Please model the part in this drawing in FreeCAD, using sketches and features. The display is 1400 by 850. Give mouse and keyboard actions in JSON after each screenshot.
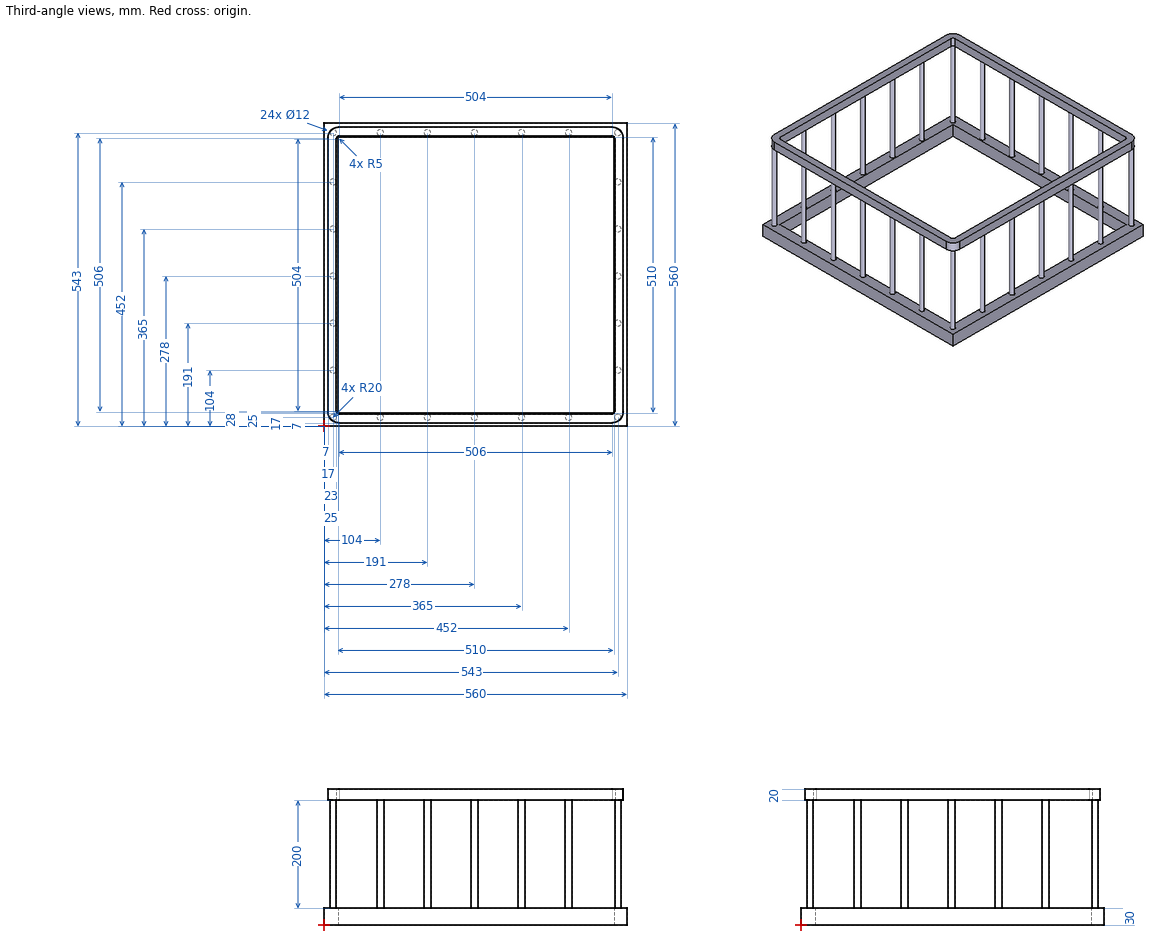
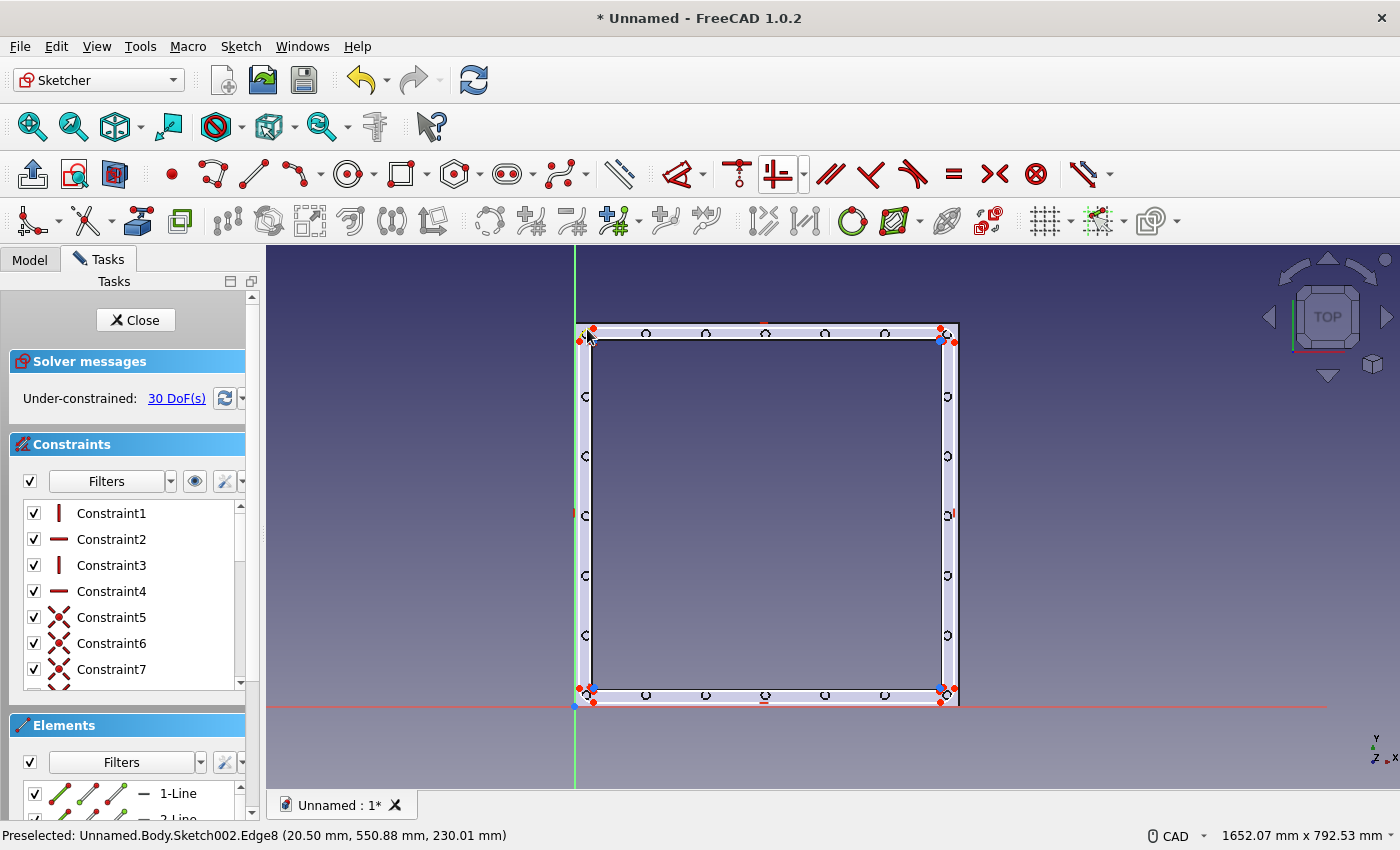
{"action": "scroll", "coordinate": [697, 703], "scroll_direction": "up", "scroll_amount": 6}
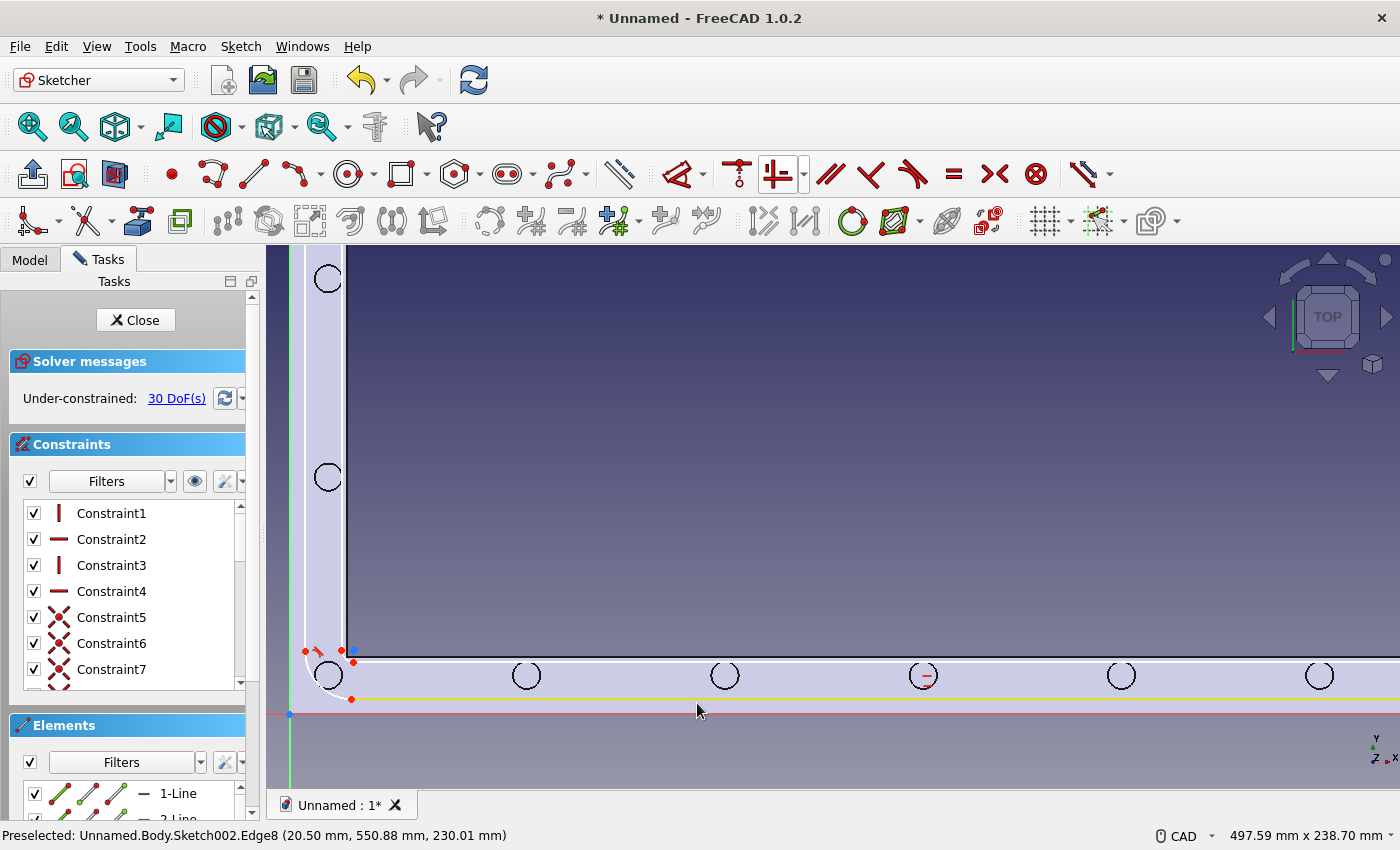
{"action": "left_click", "coordinate": [697, 699]}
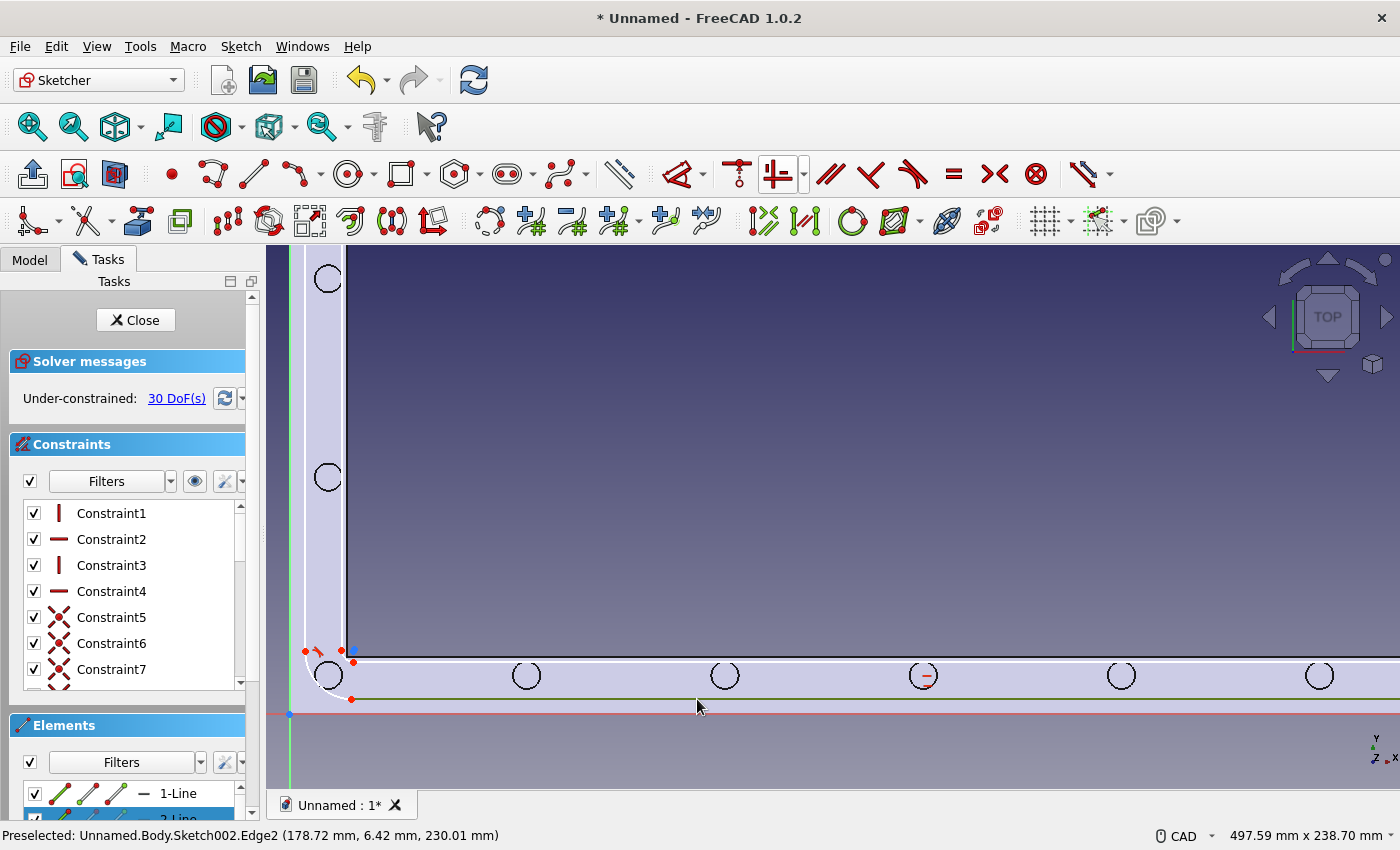
{"action": "left_click", "coordinate": [310, 673]}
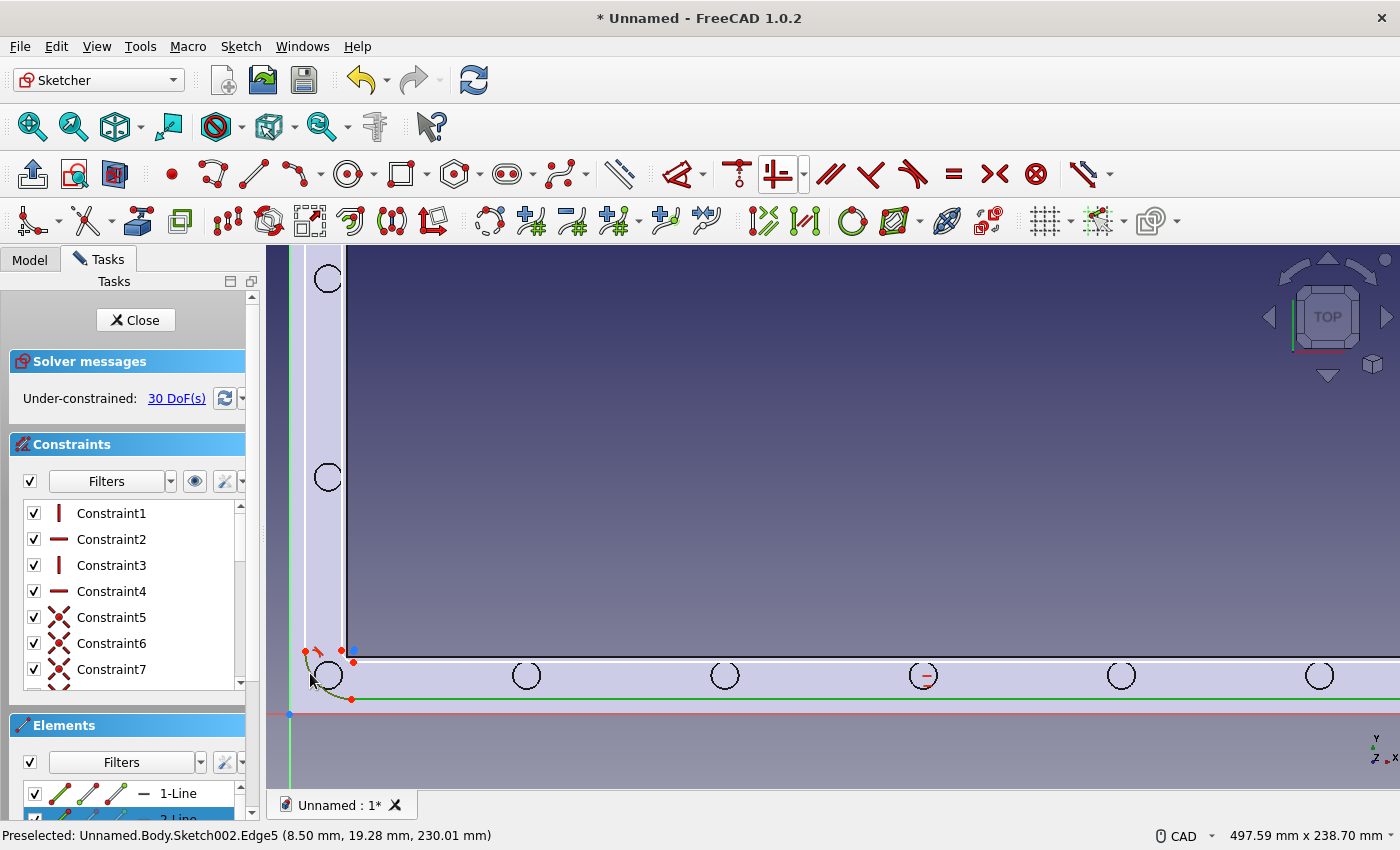
{"action": "left_click", "coordinate": [913, 174]}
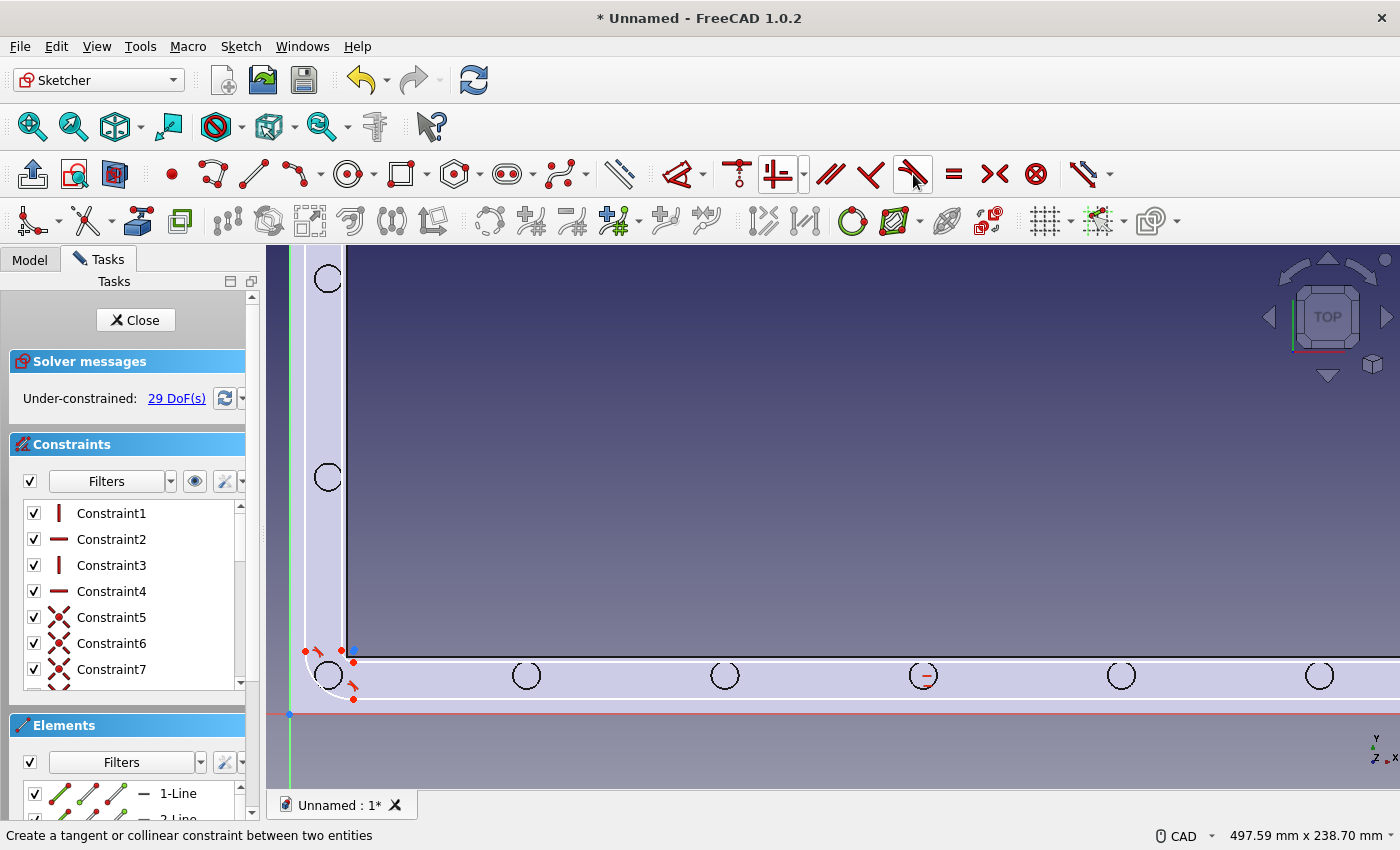
{"action": "left_click", "coordinate": [699, 699]}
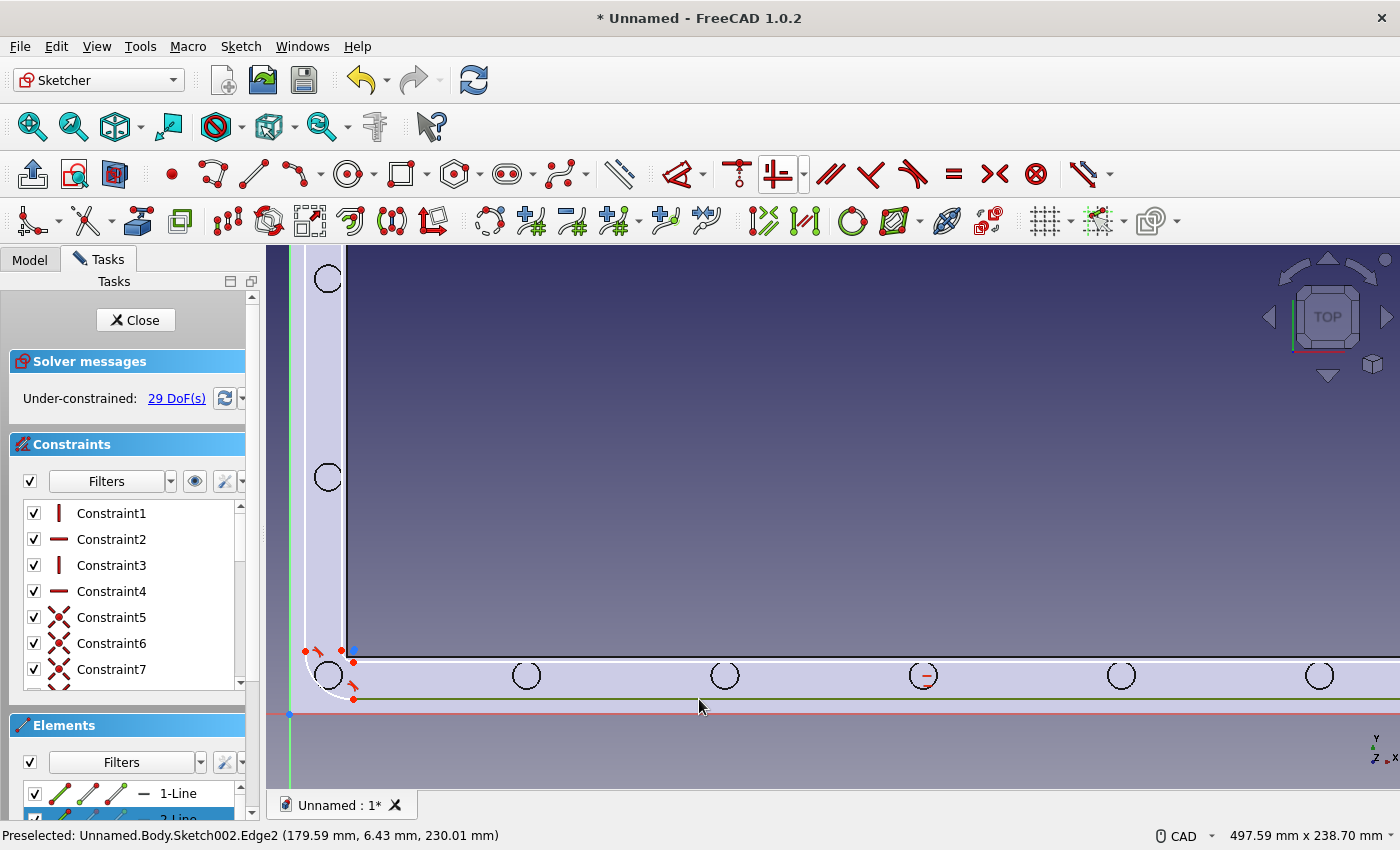
{"action": "scroll", "coordinate": [698, 704], "scroll_direction": "down", "scroll_amount": 6}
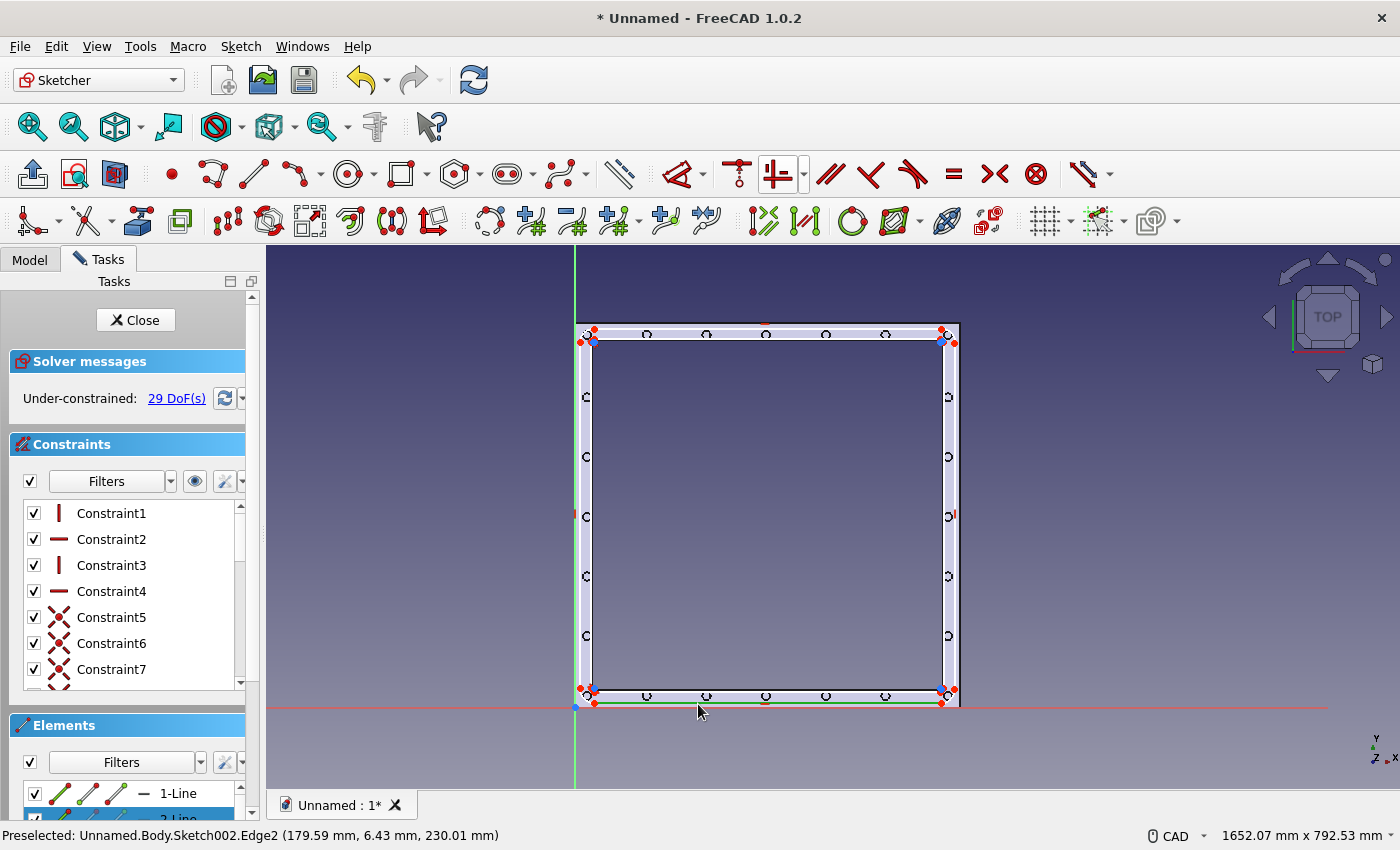
{"action": "scroll", "coordinate": [947, 702], "scroll_direction": "up", "scroll_amount": 5}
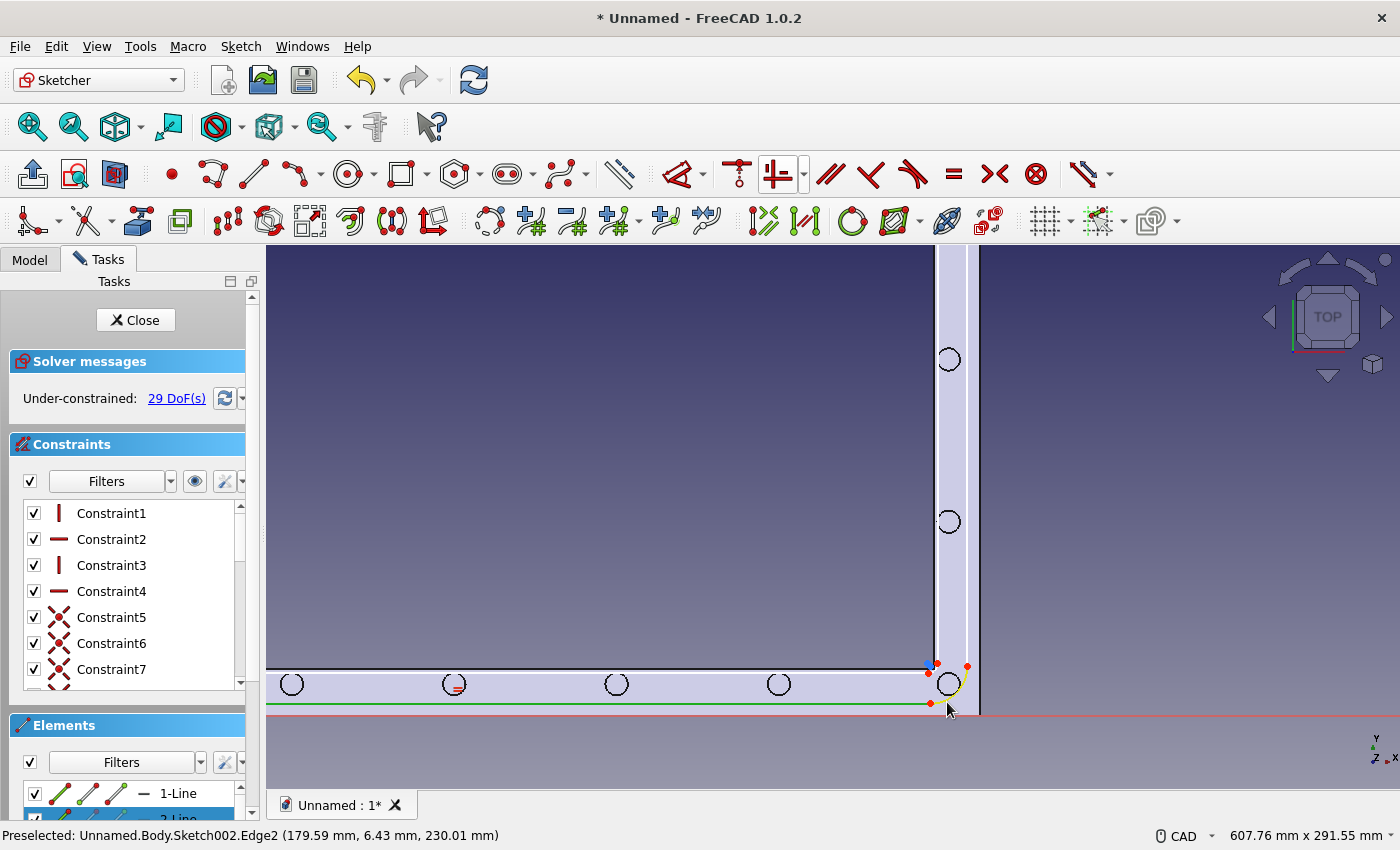
{"action": "left_click", "coordinate": [947, 700]}